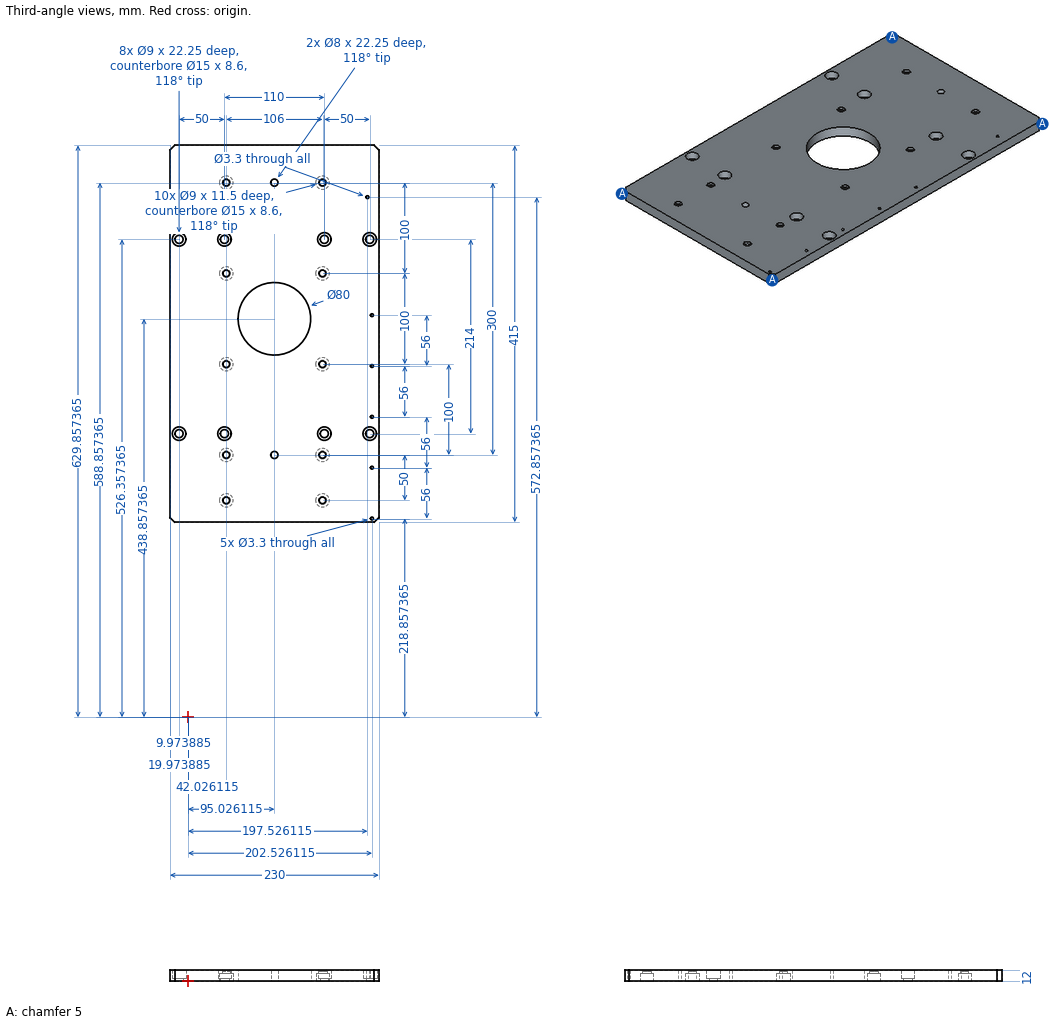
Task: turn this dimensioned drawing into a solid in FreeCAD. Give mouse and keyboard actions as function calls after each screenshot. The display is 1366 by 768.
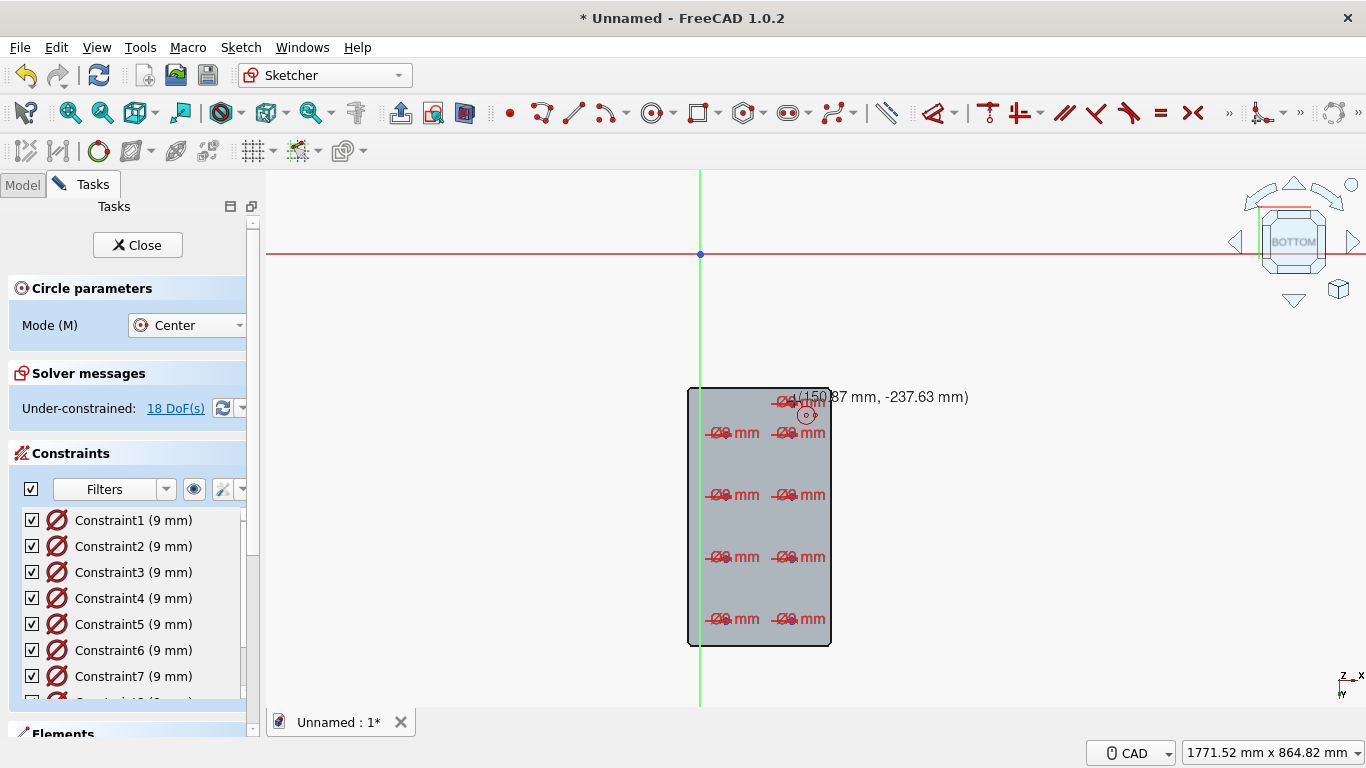
scroll(726, 403, up, 11)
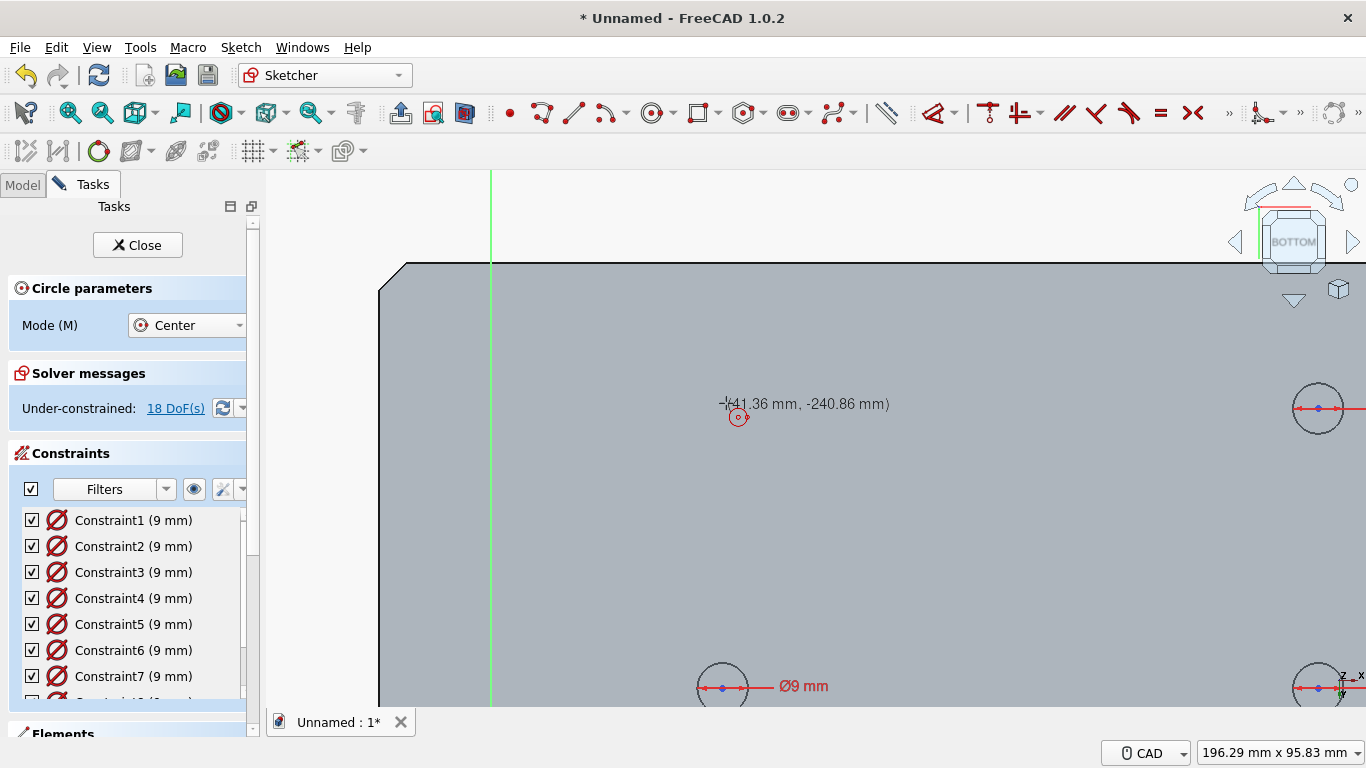
scroll(726, 403, down, 11)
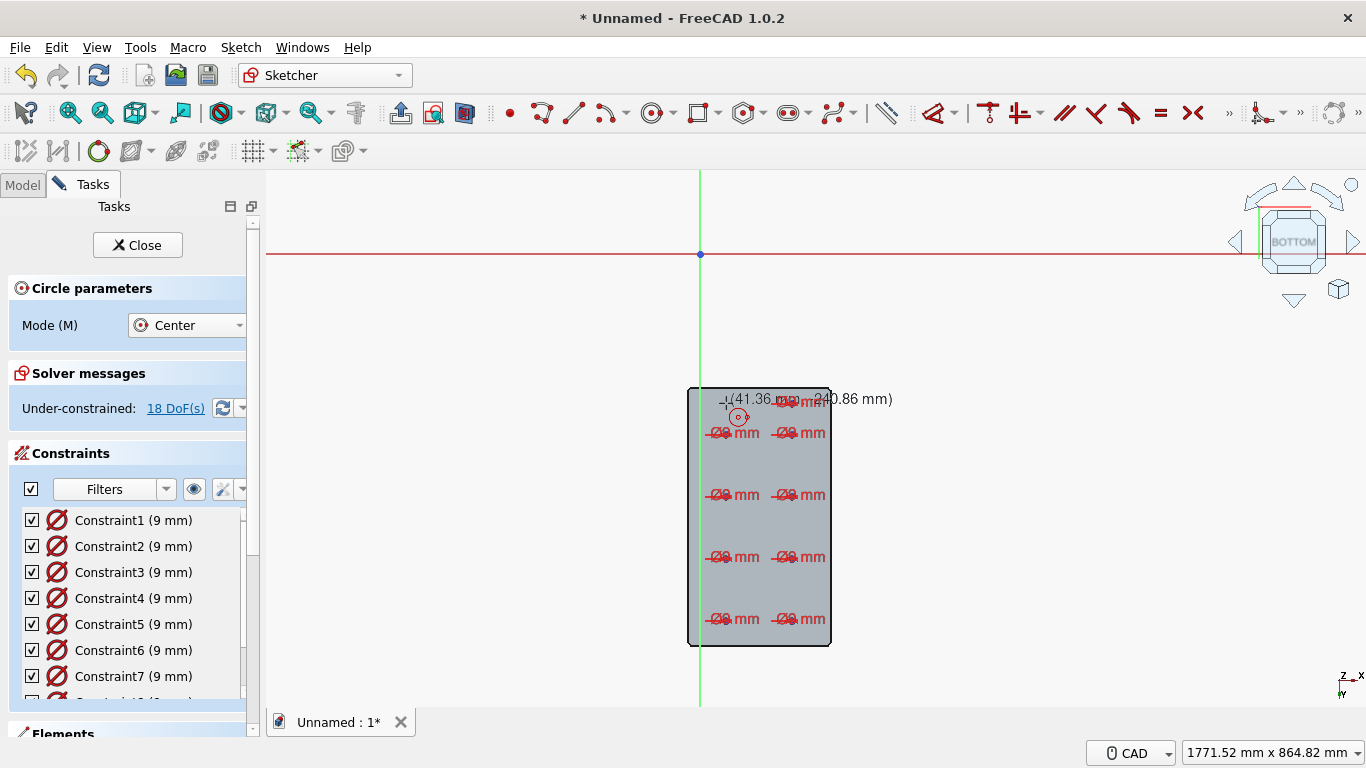
click(726, 403)
move(728, 401)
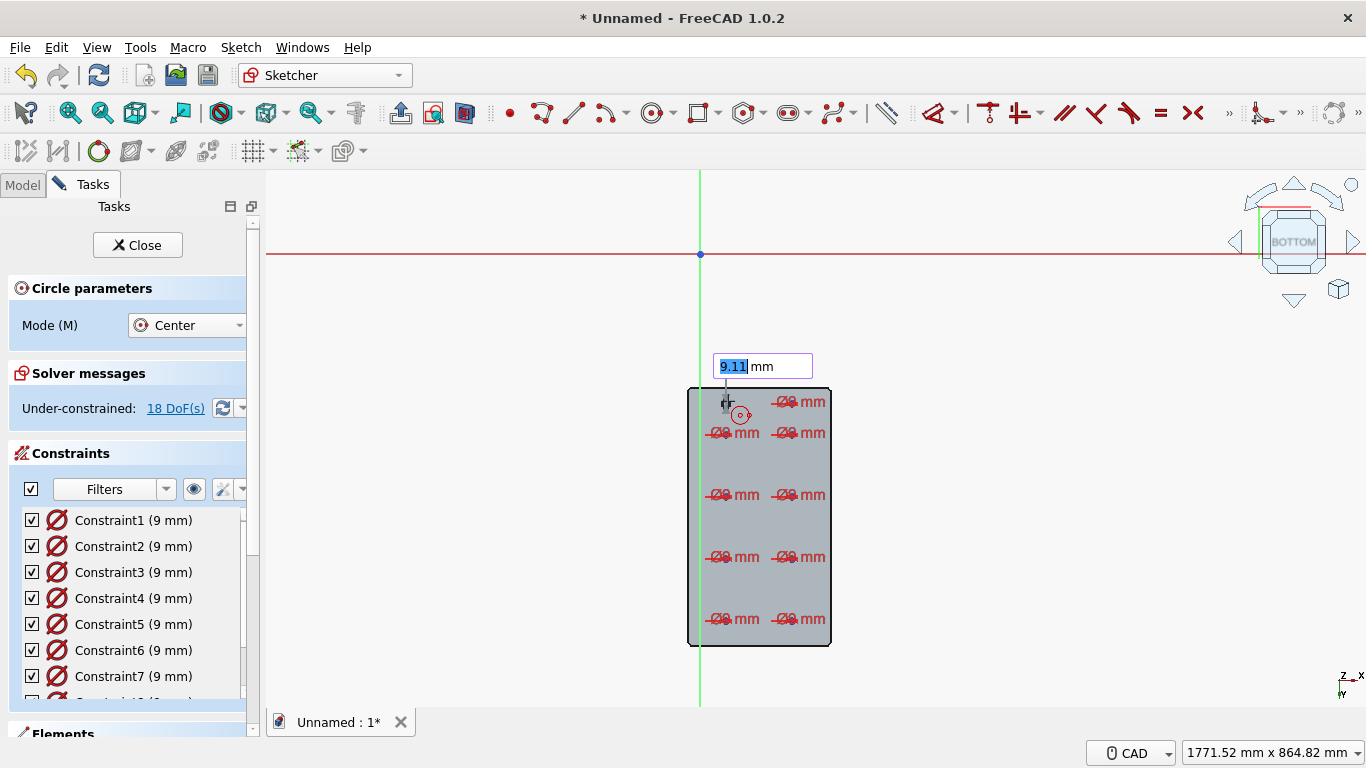
text(9)
key(Return)
key(Escape)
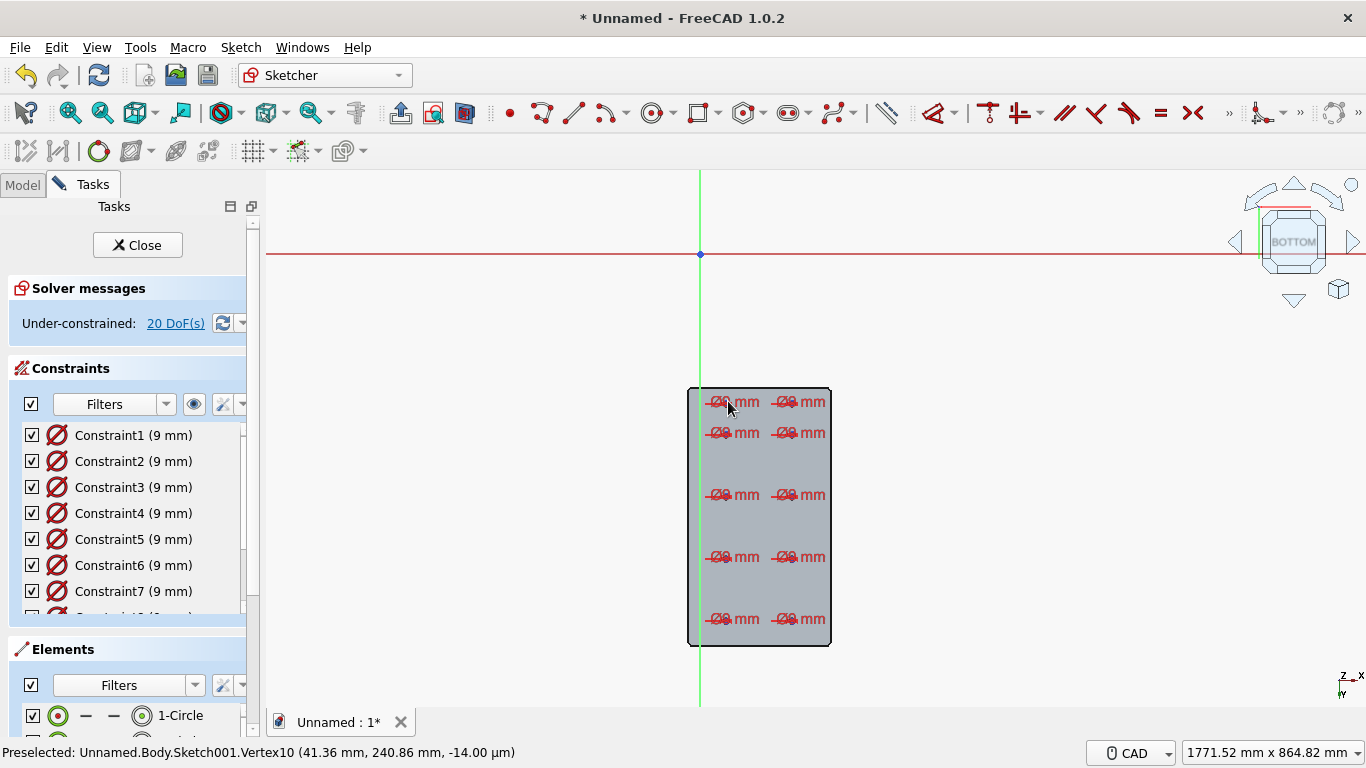
click(792, 621)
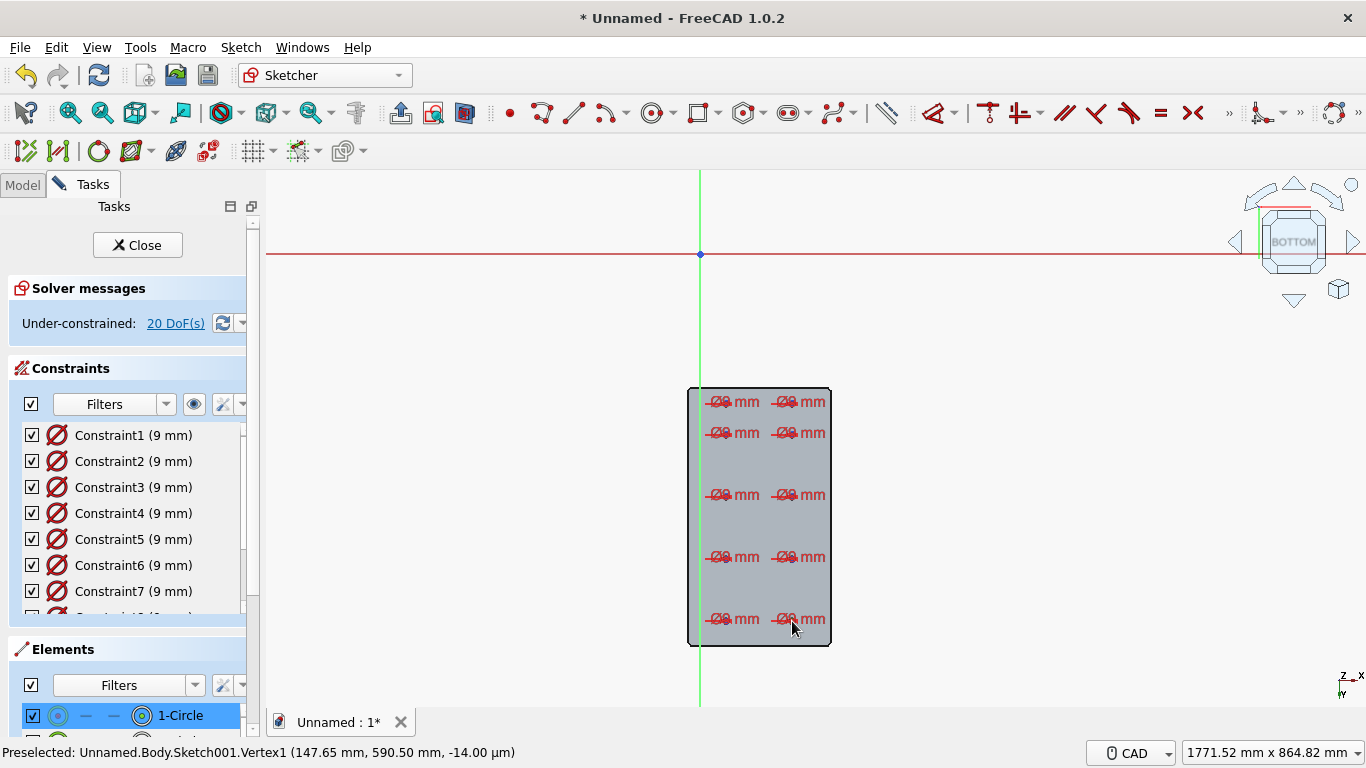
click(726, 621)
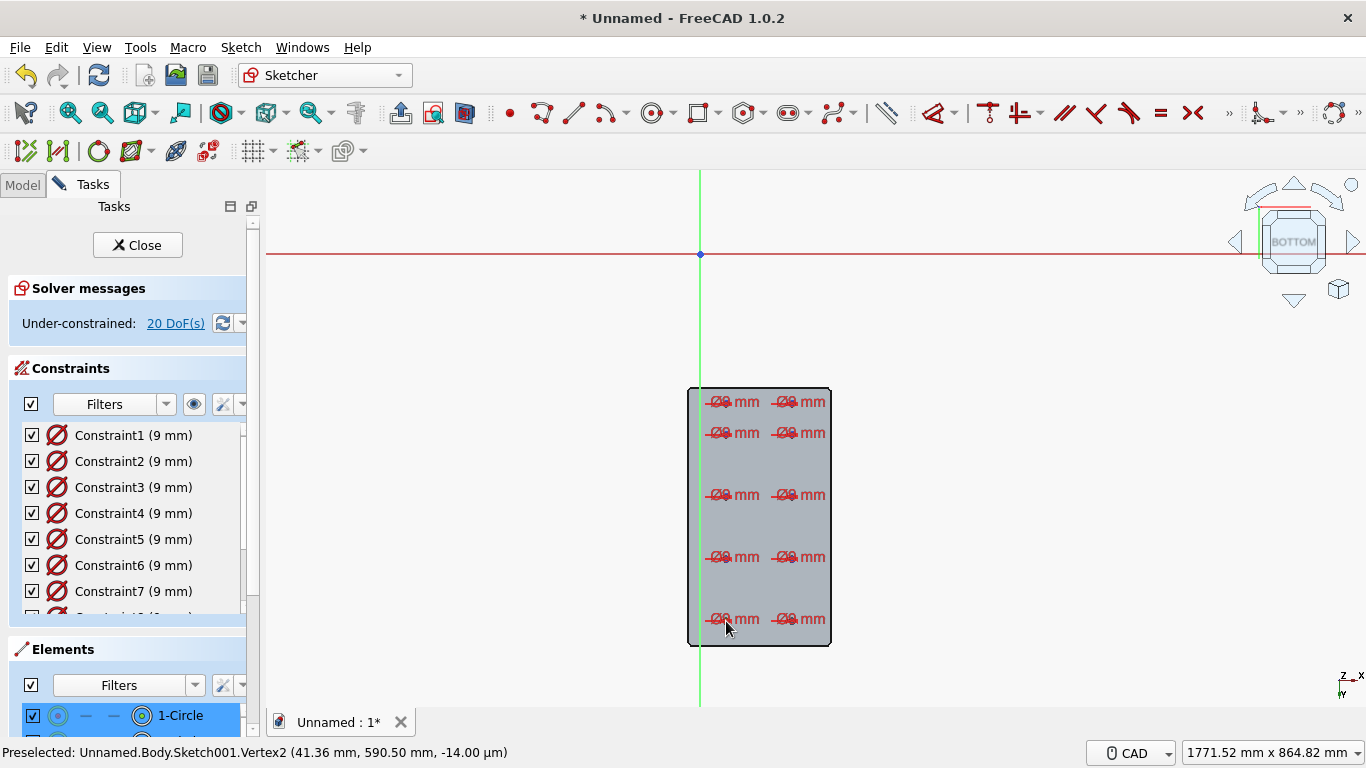
click(1042, 114)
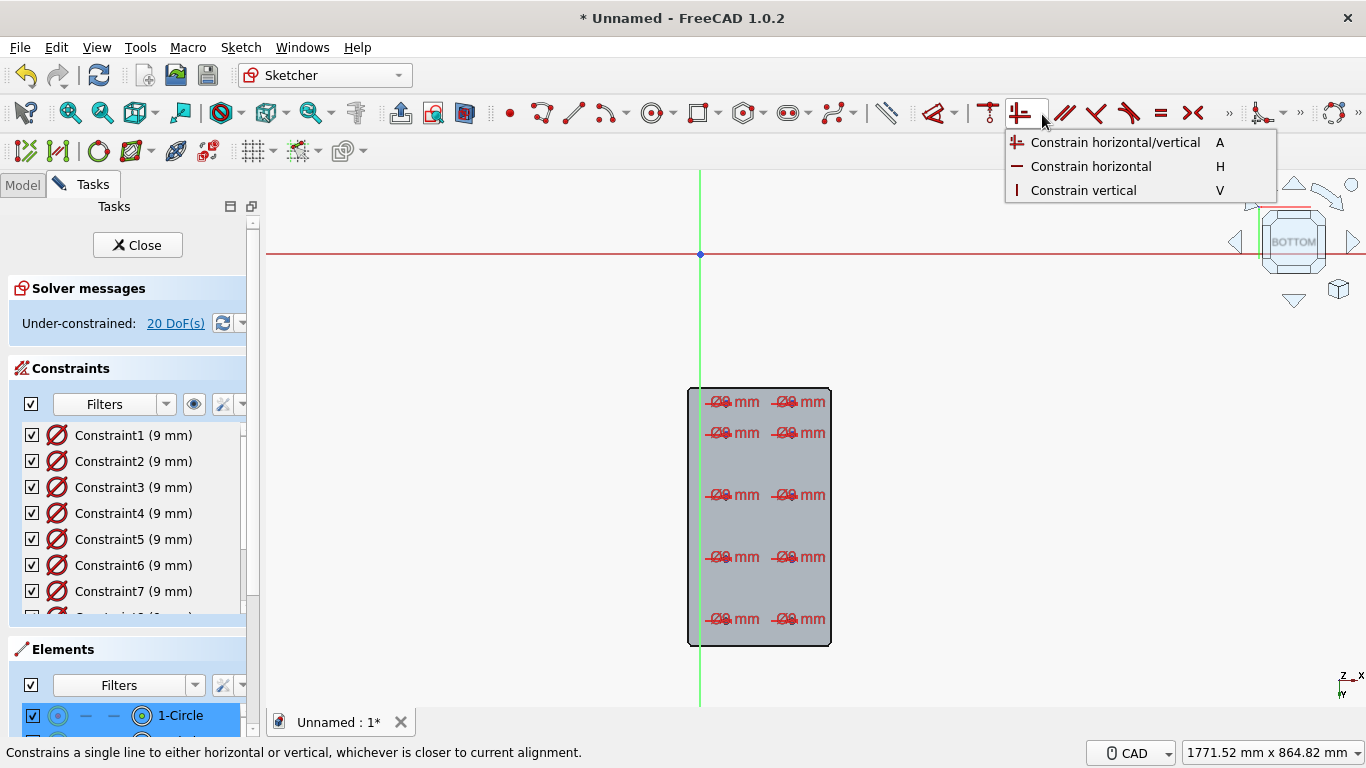
click(1141, 166)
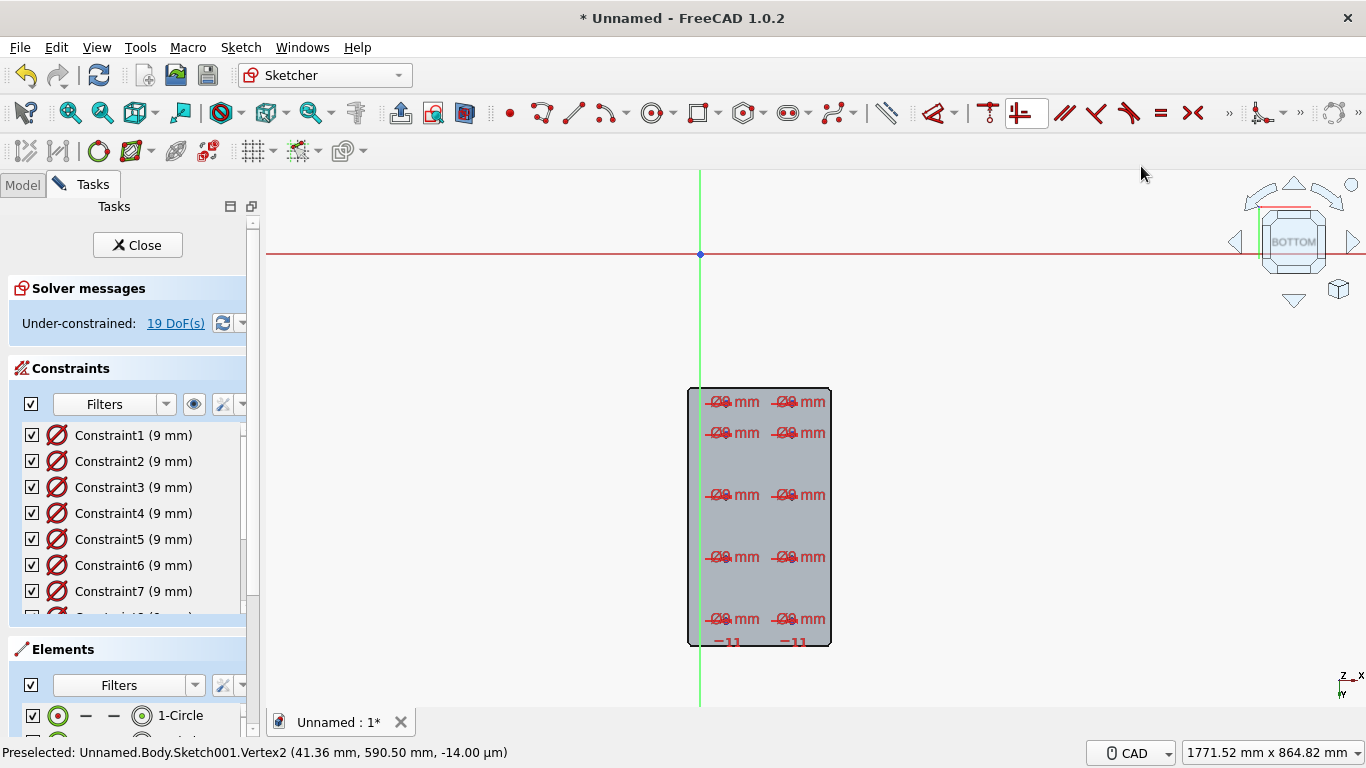
click(792, 621)